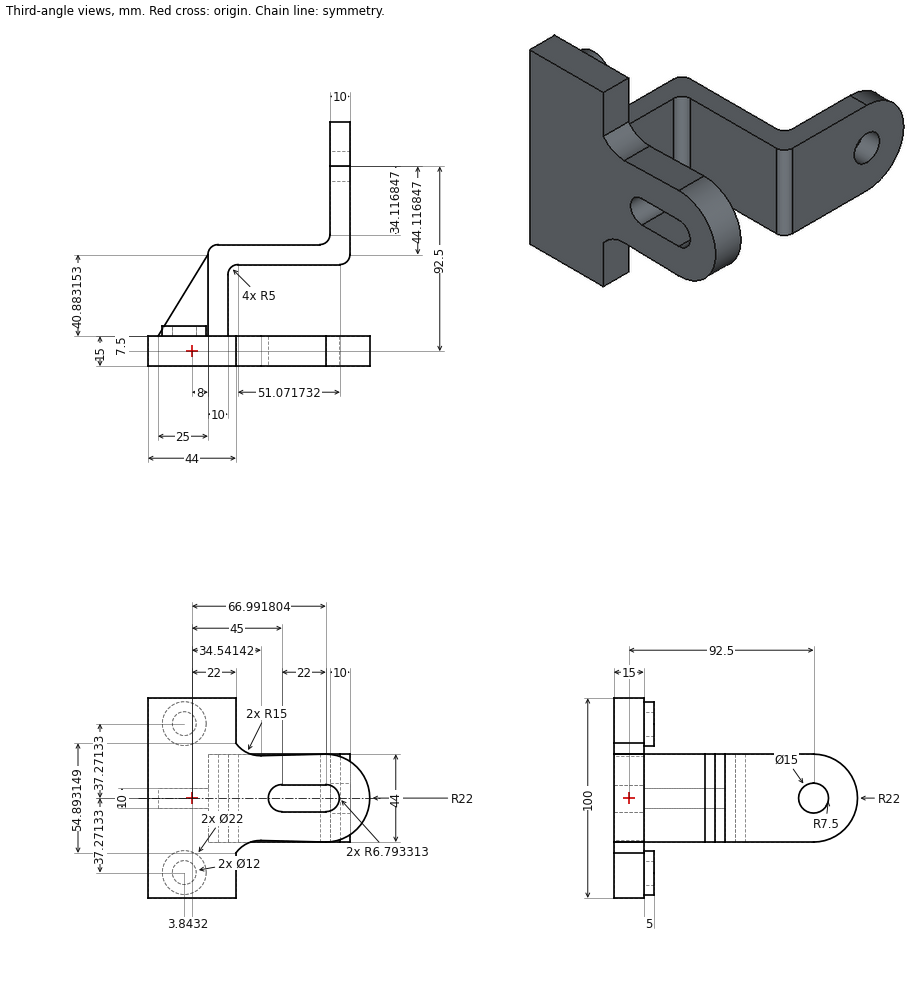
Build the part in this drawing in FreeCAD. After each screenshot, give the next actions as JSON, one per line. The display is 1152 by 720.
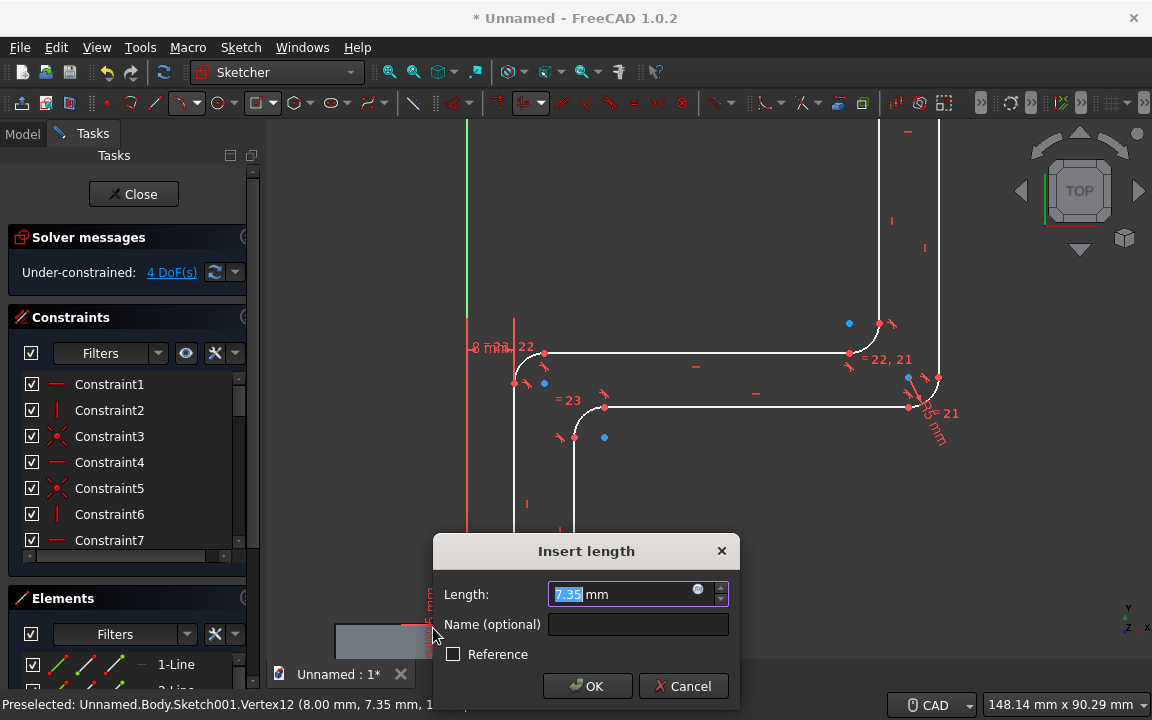
{"action": "type", "text": "7.5"}
{"action": "key", "text": "Return"}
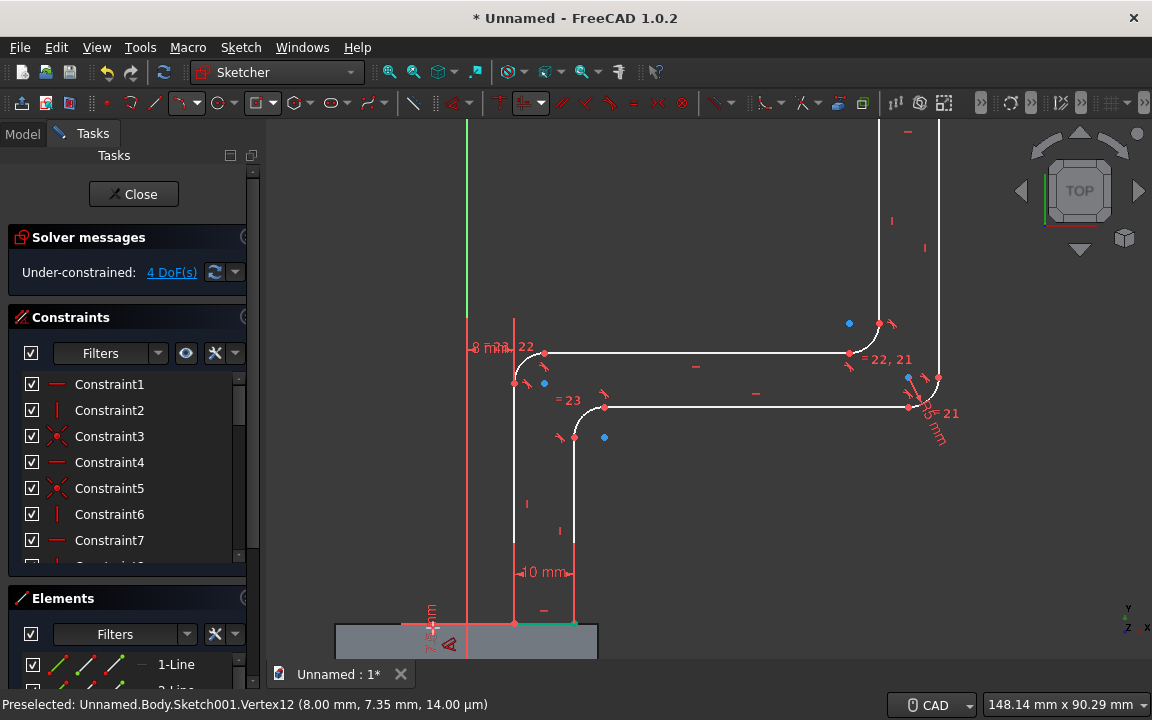
{"action": "scroll", "coordinate": [513, 383], "scroll_direction": "down", "scroll_amount": 2}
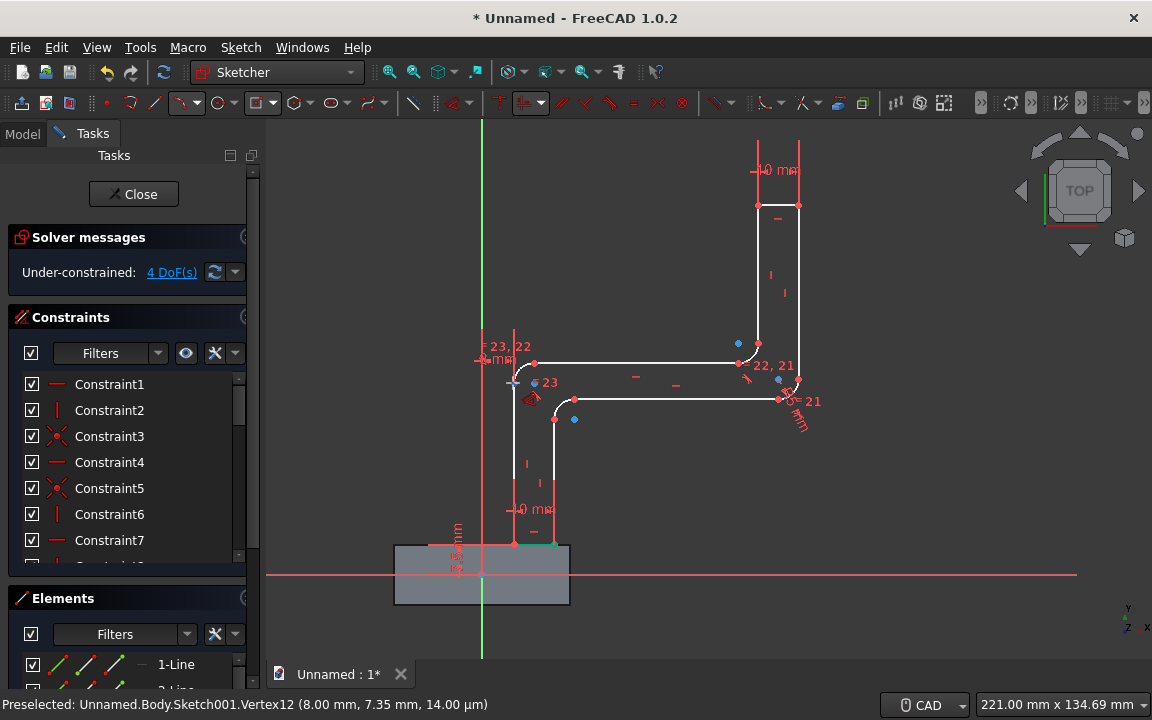
{"action": "left_click", "coordinate": [799, 205]}
{"action": "left_click", "coordinate": [448, 390]}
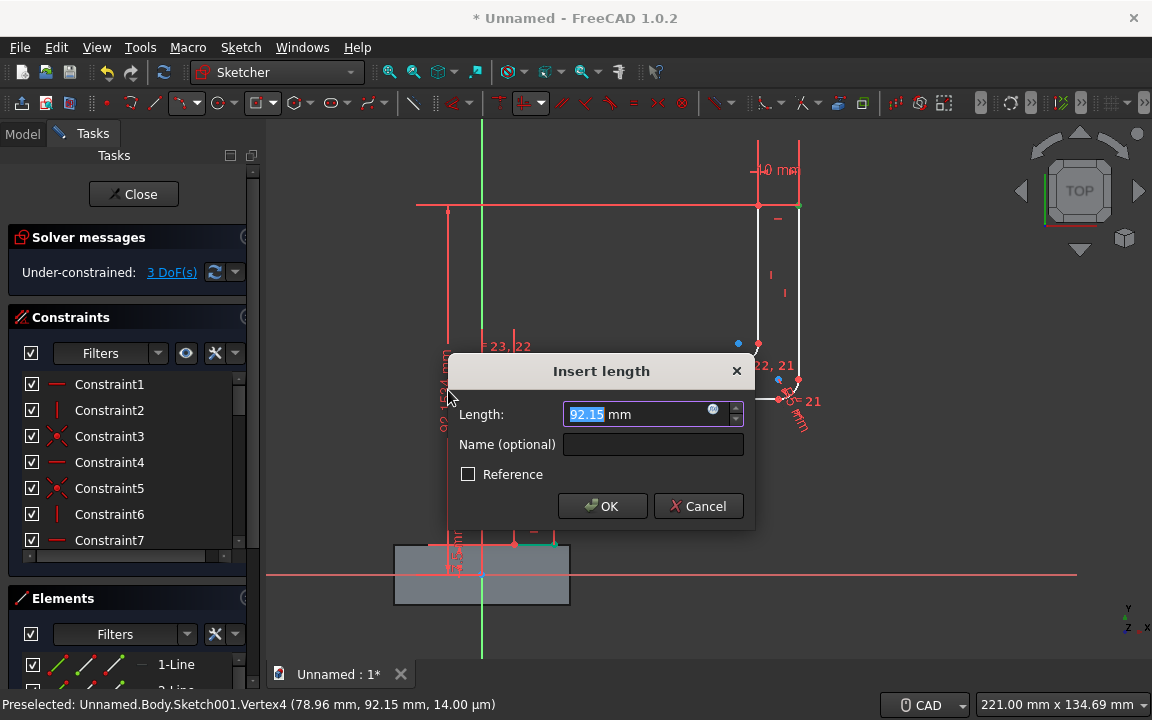
{"action": "type", "text": "92.5"}
{"action": "key", "text": "Return"}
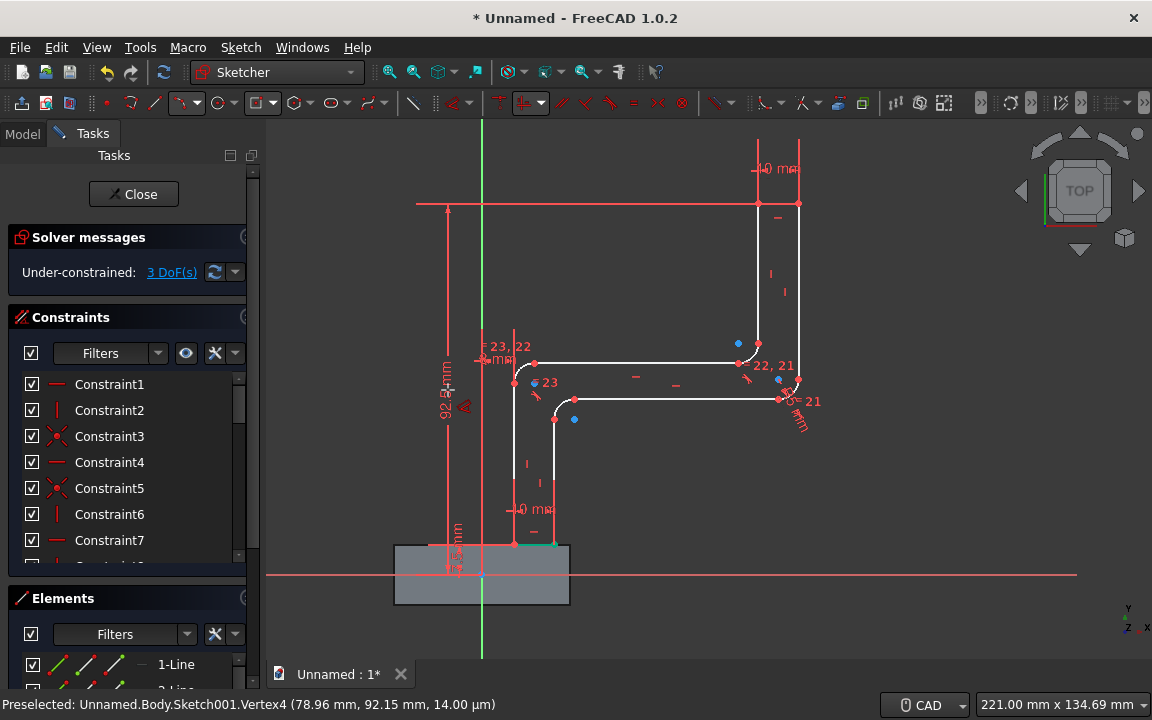
{"action": "left_click", "coordinate": [635, 399]}
{"action": "left_click", "coordinate": [676, 433]}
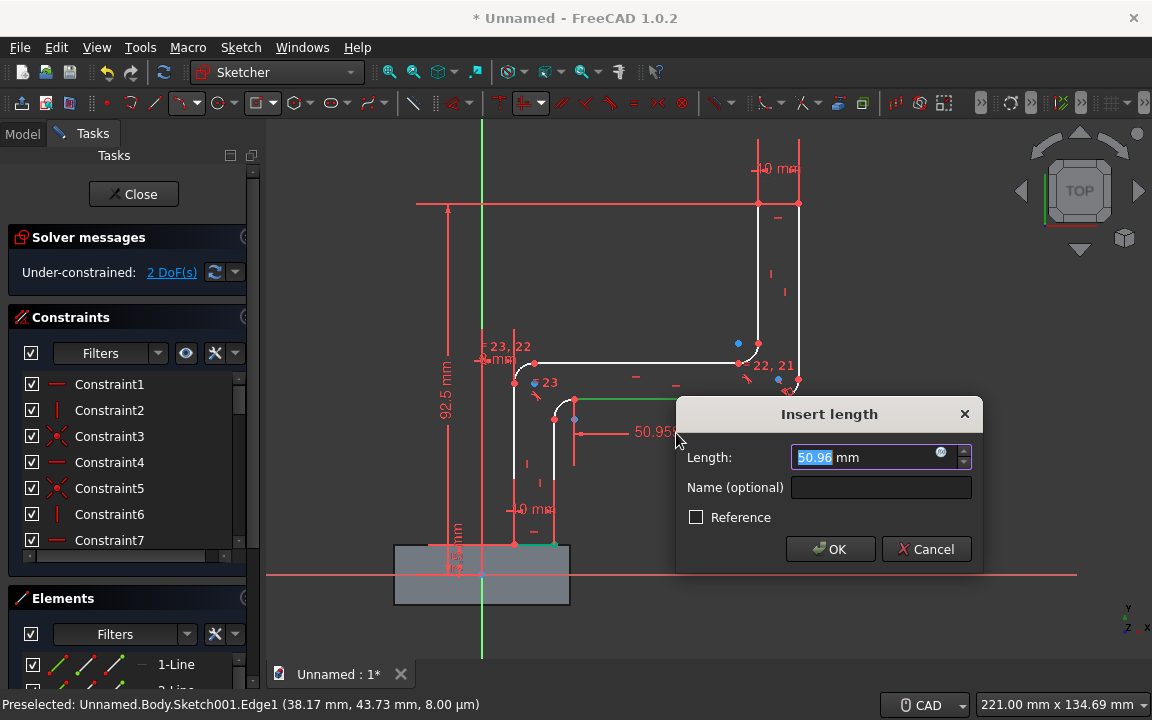
{"action": "type", "text": "51.071732"}
{"action": "key", "text": "Return"}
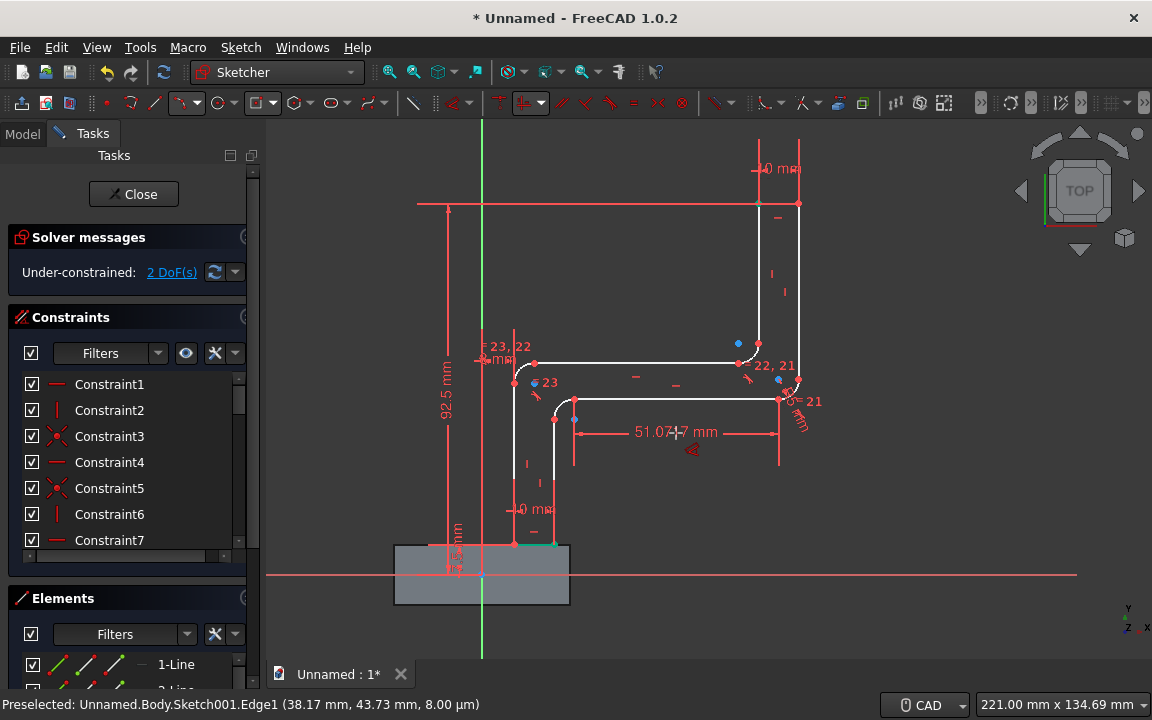
{"action": "left_click", "coordinate": [799, 327]}
{"action": "left_click", "coordinate": [833, 292]}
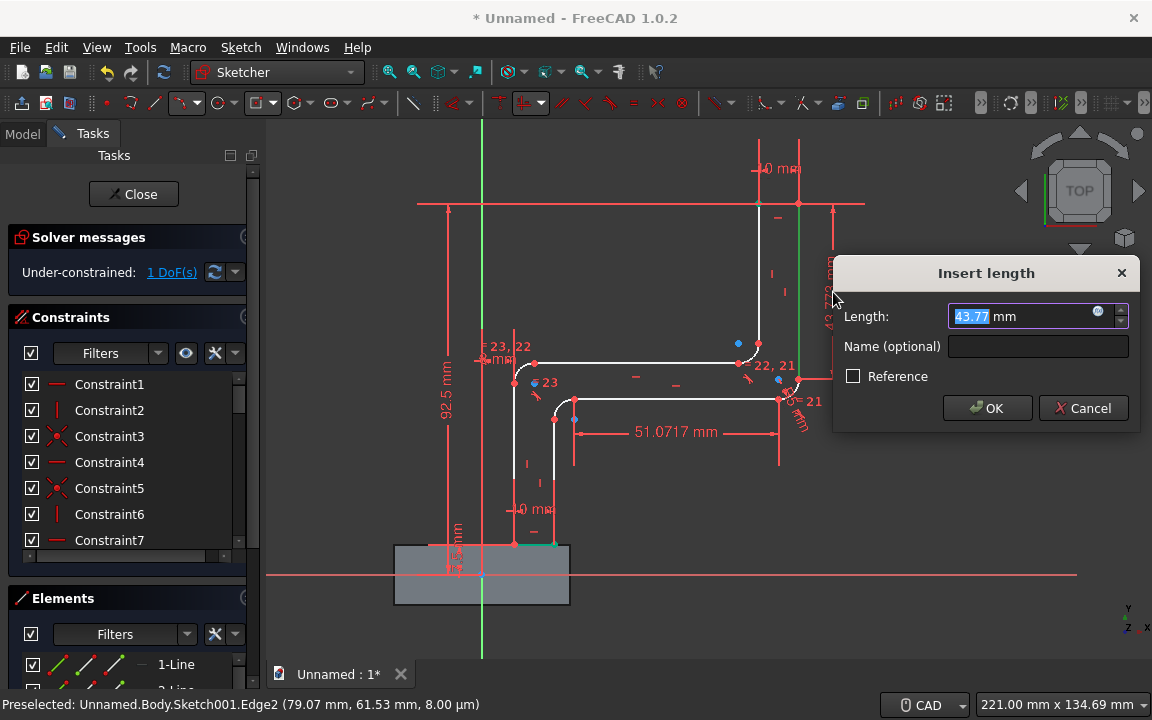
{"action": "type", "text": "44.116847"}
{"action": "key", "text": "Return"}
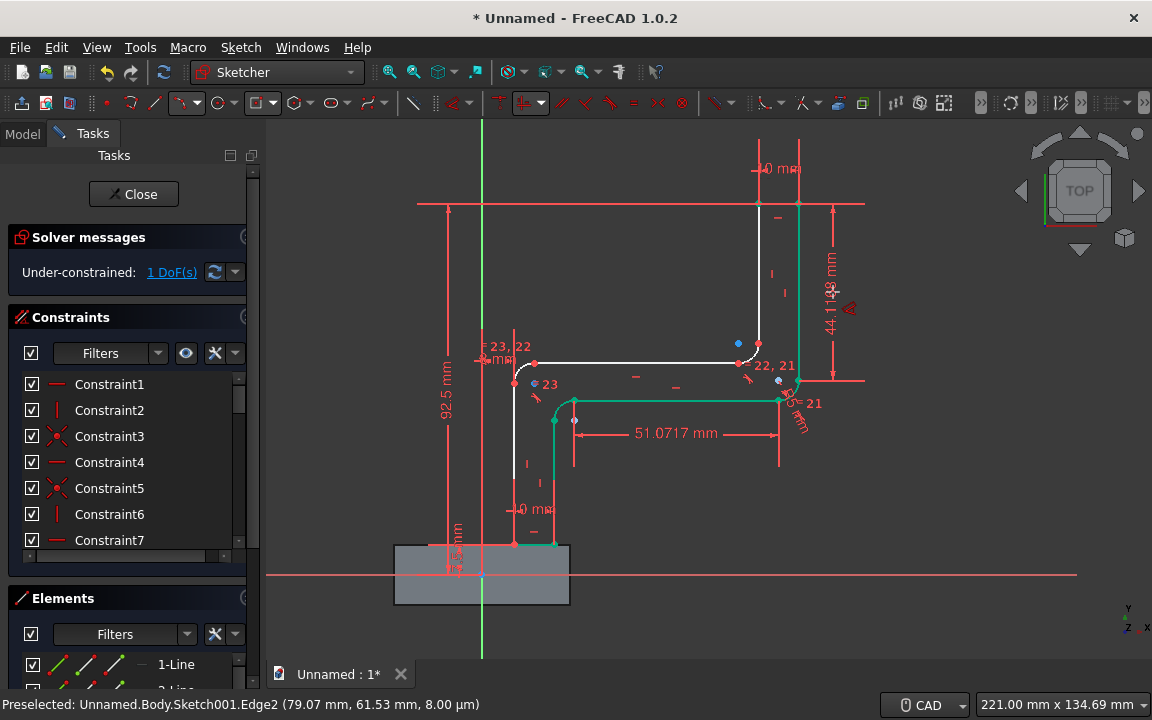
{"action": "left_click", "coordinate": [759, 246]}
{"action": "left_click", "coordinate": [725, 273]}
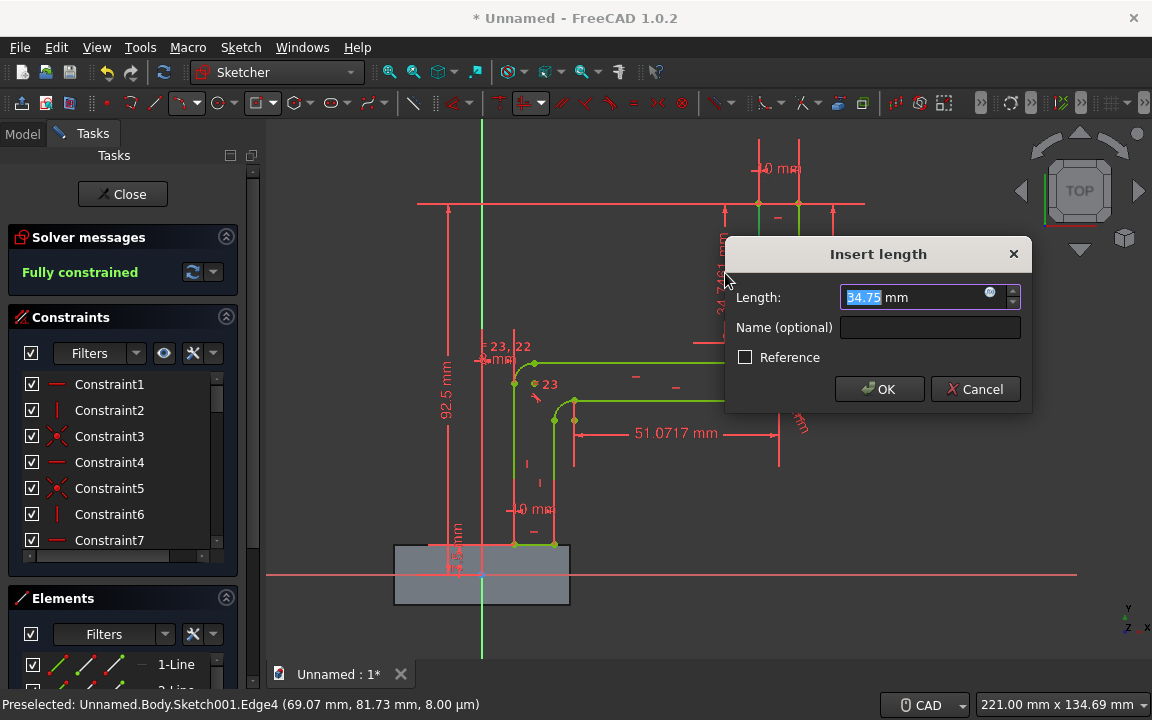
{"action": "type", "text": "34.116847"}
{"action": "key", "text": "Return"}
{"action": "key", "text": "Escape"}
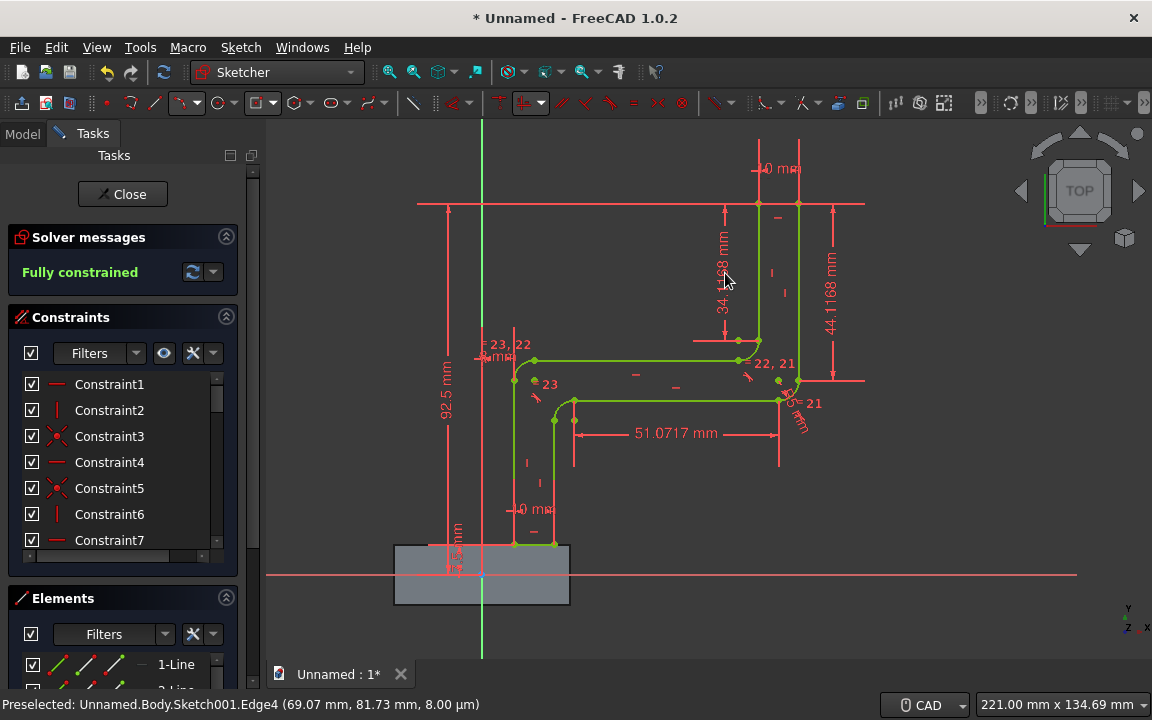
{"action": "left_click", "coordinate": [123, 194]}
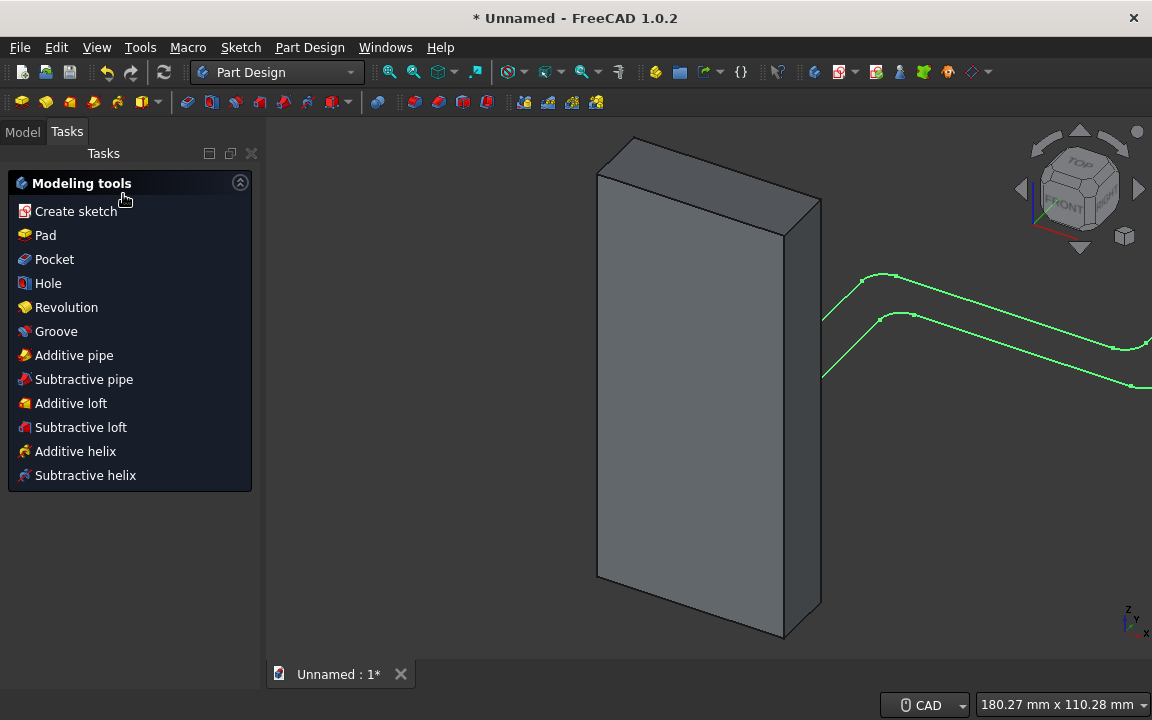
{"action": "left_click", "coordinate": [22, 102]}